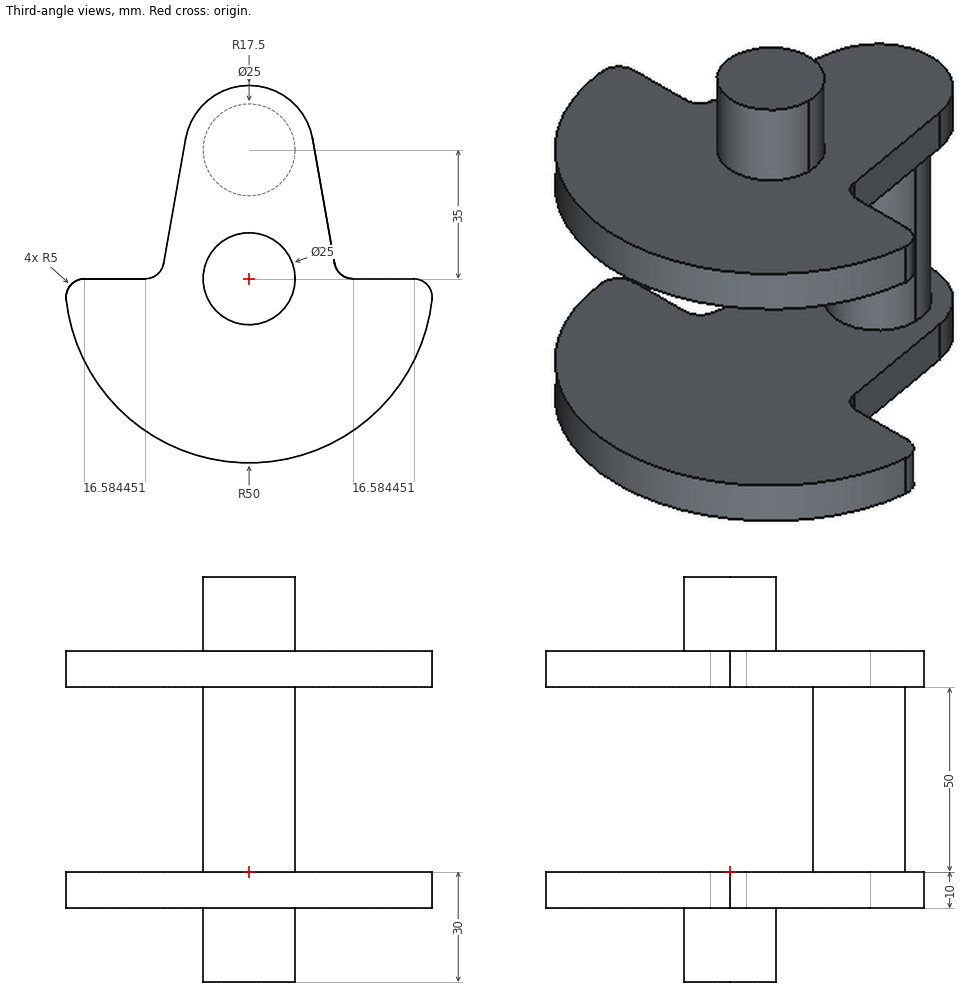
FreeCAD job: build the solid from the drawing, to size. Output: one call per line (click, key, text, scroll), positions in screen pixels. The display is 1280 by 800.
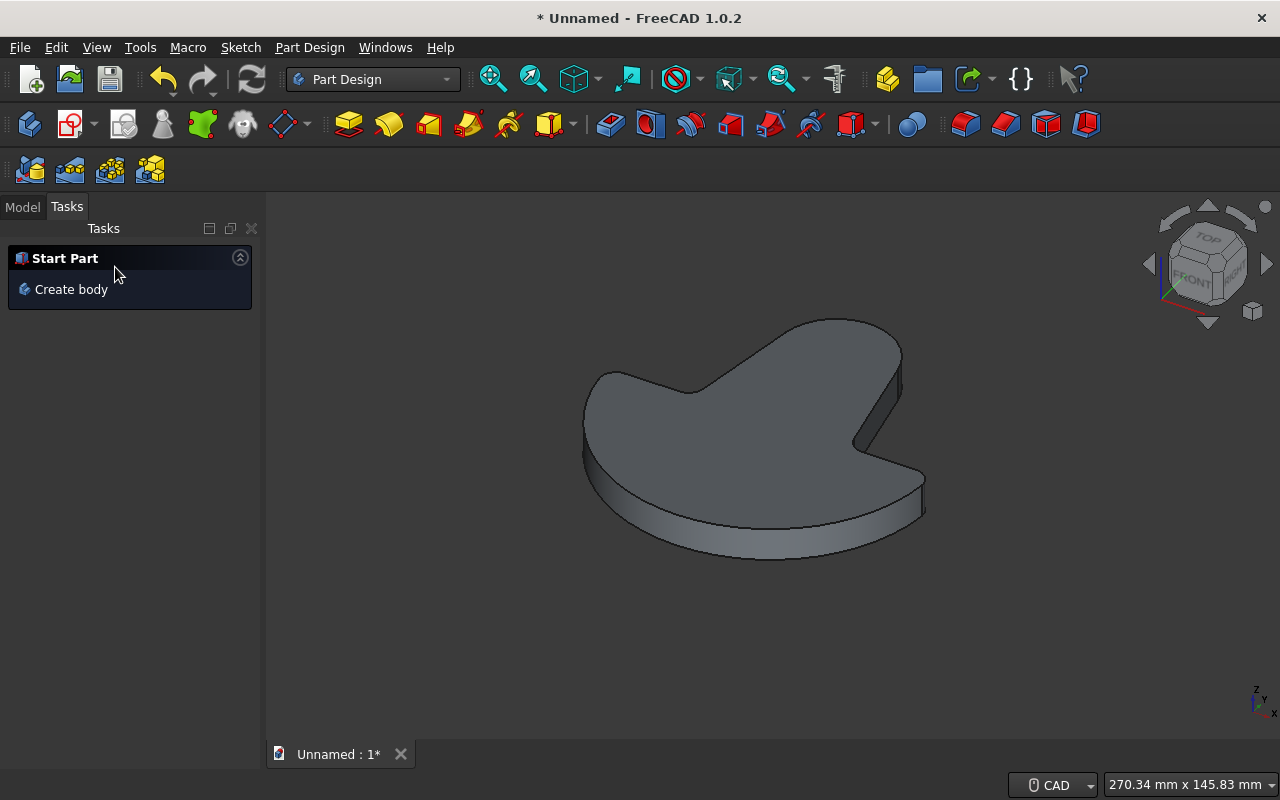
click(70, 124)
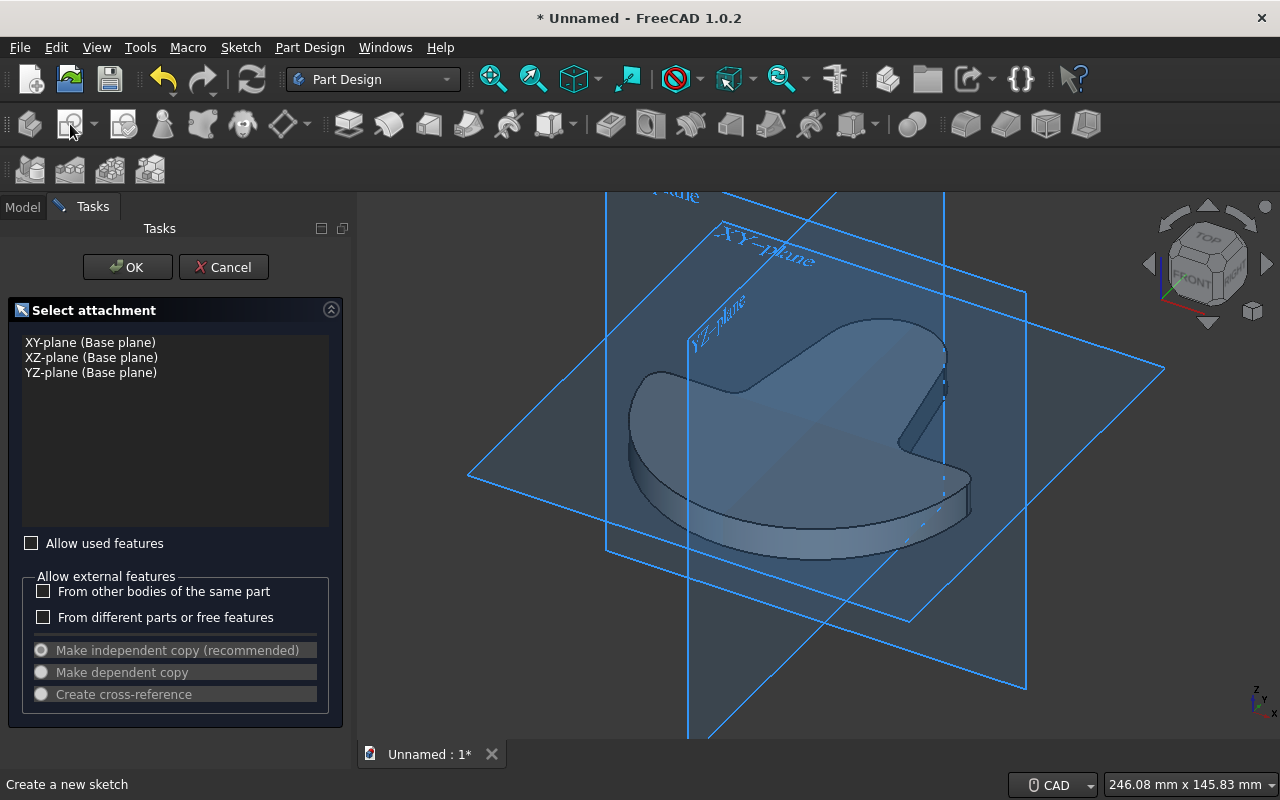
click(82, 342)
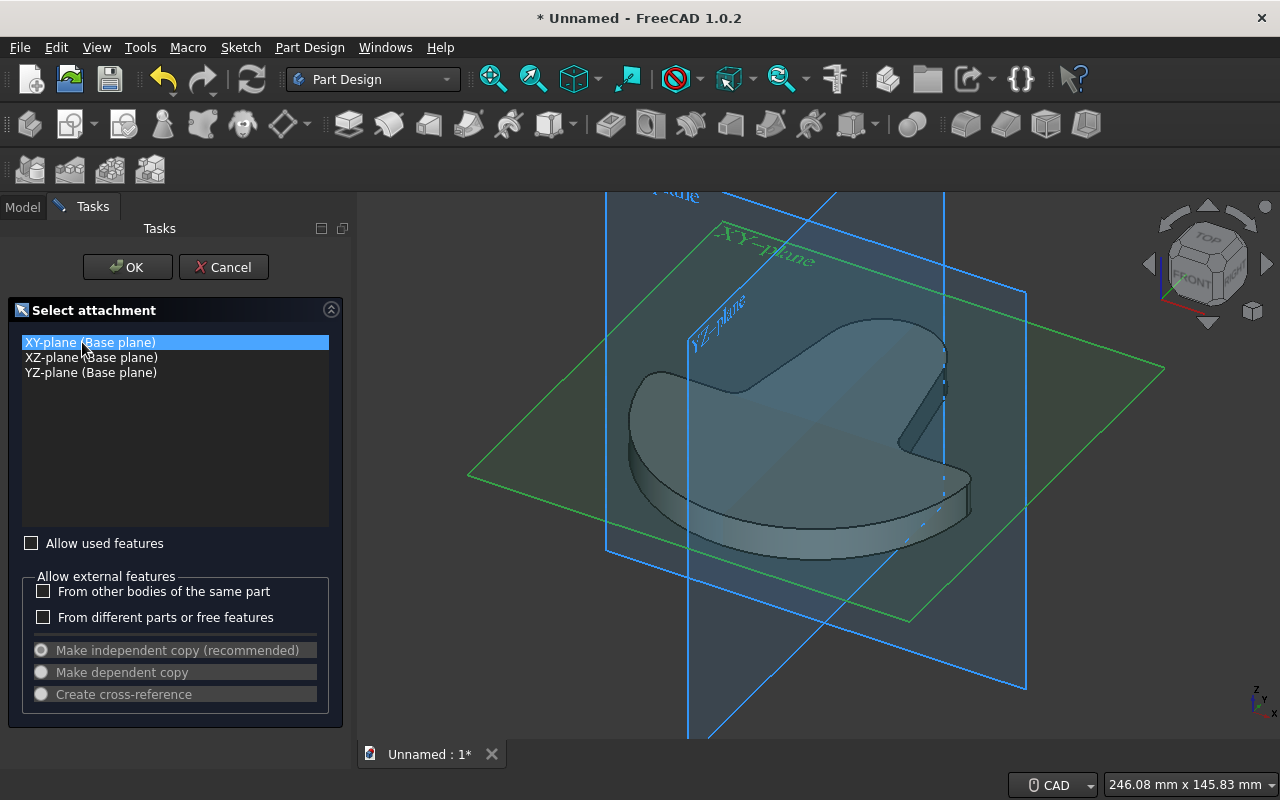
click(128, 267)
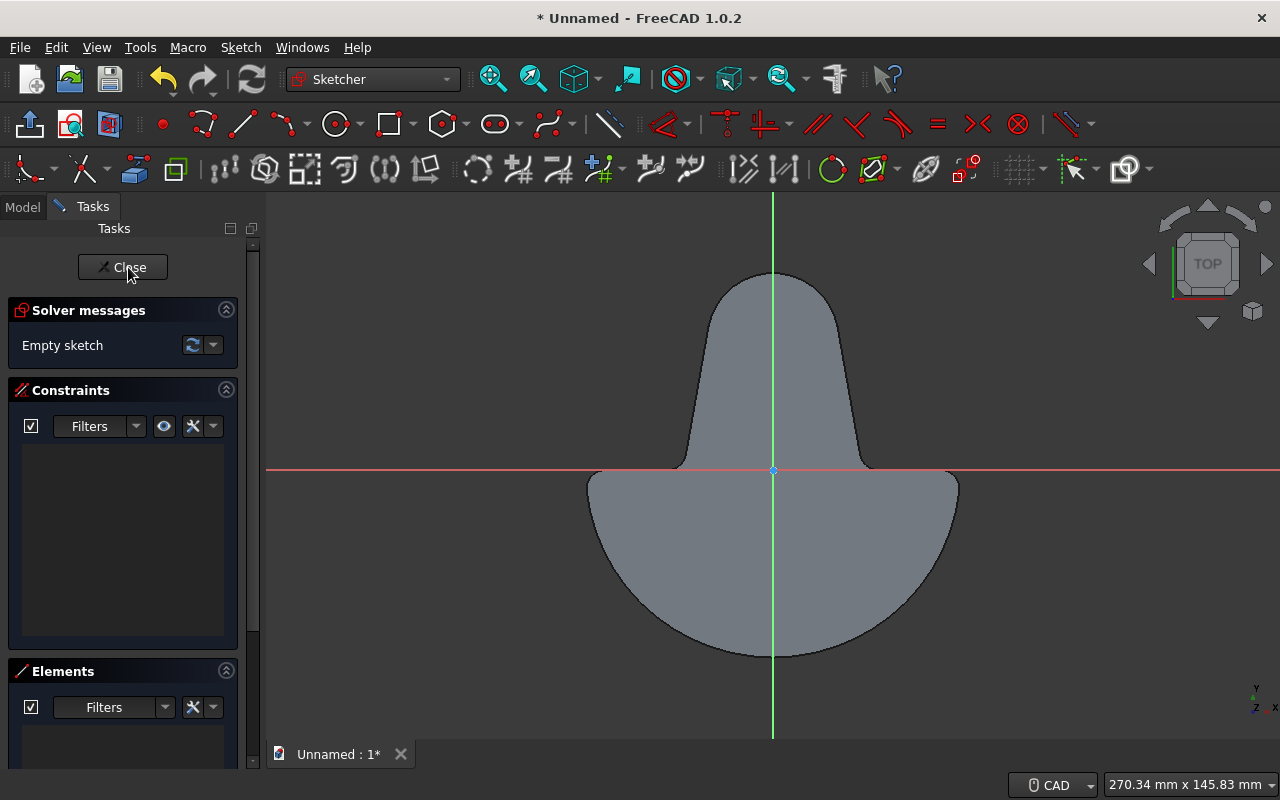
scroll(856, 278, up, 3)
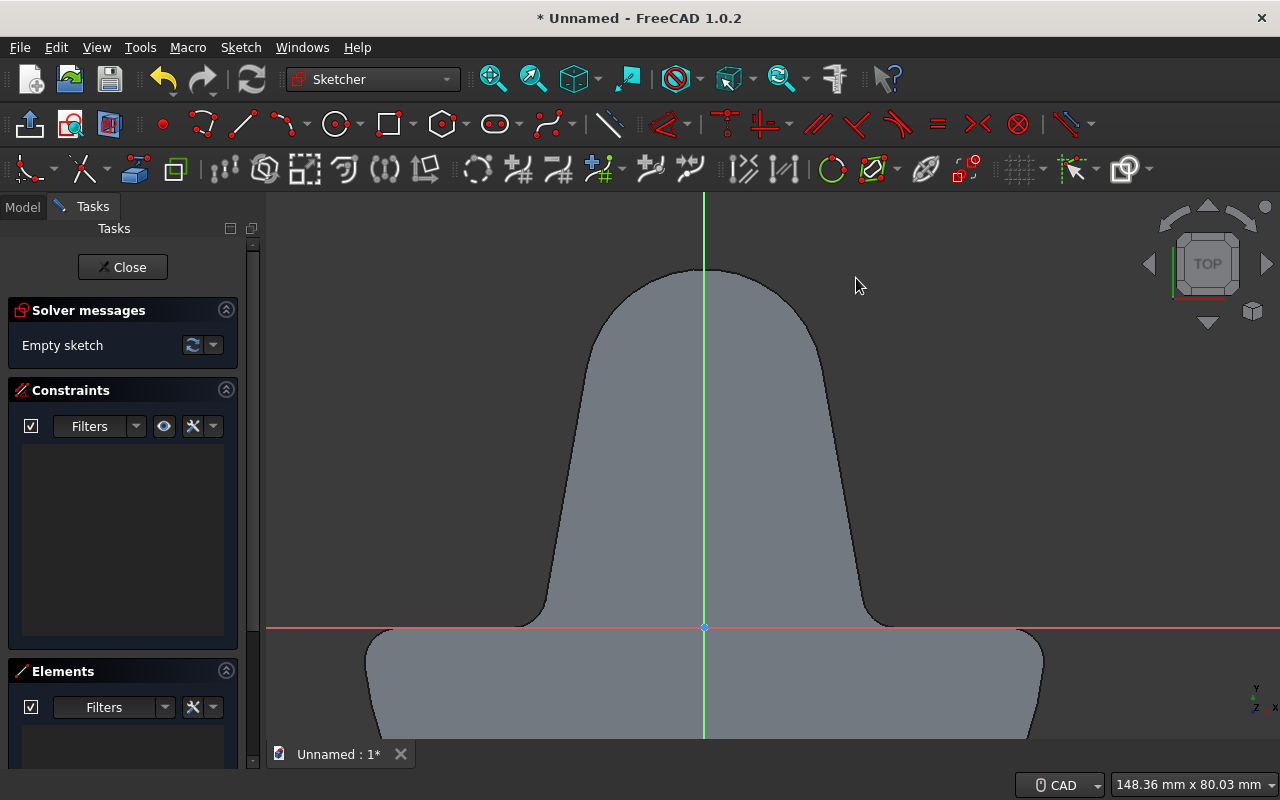
key(g)
key(c)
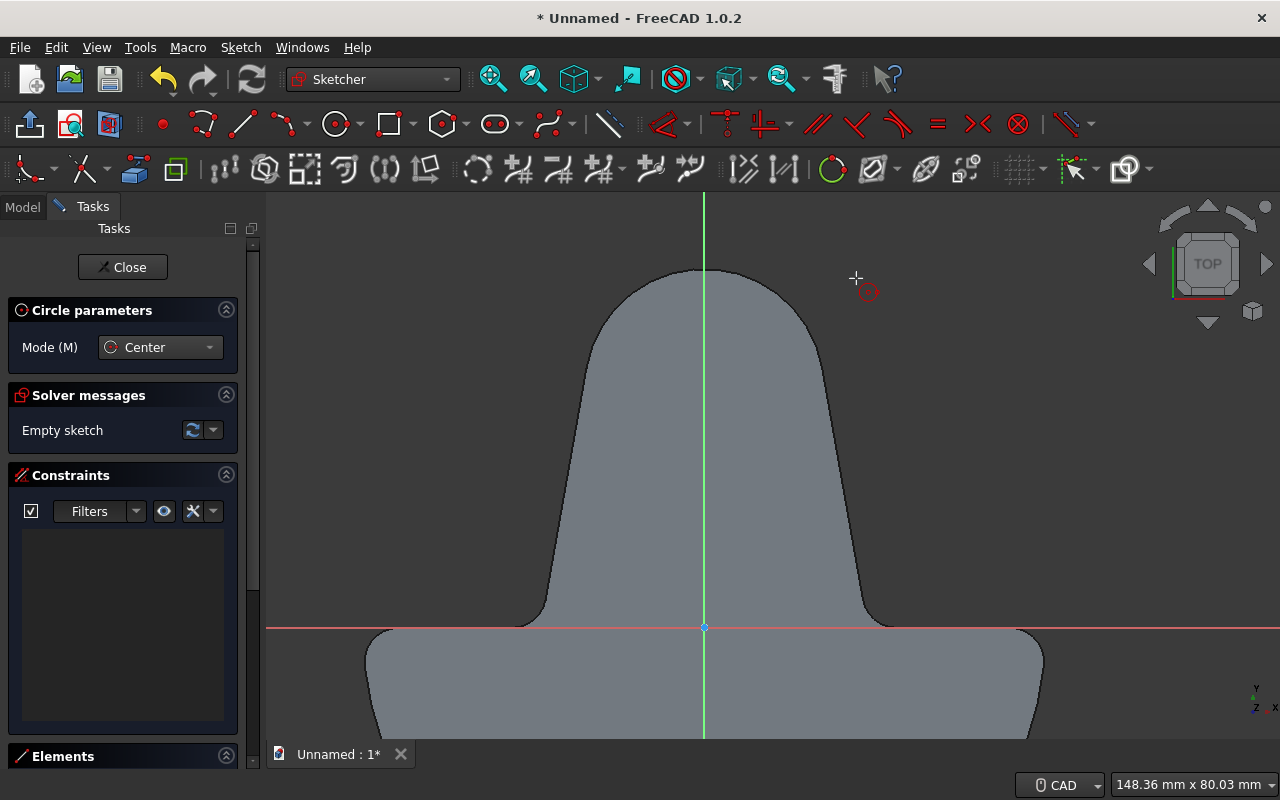
click(704, 389)
click(765, 328)
key(Escape)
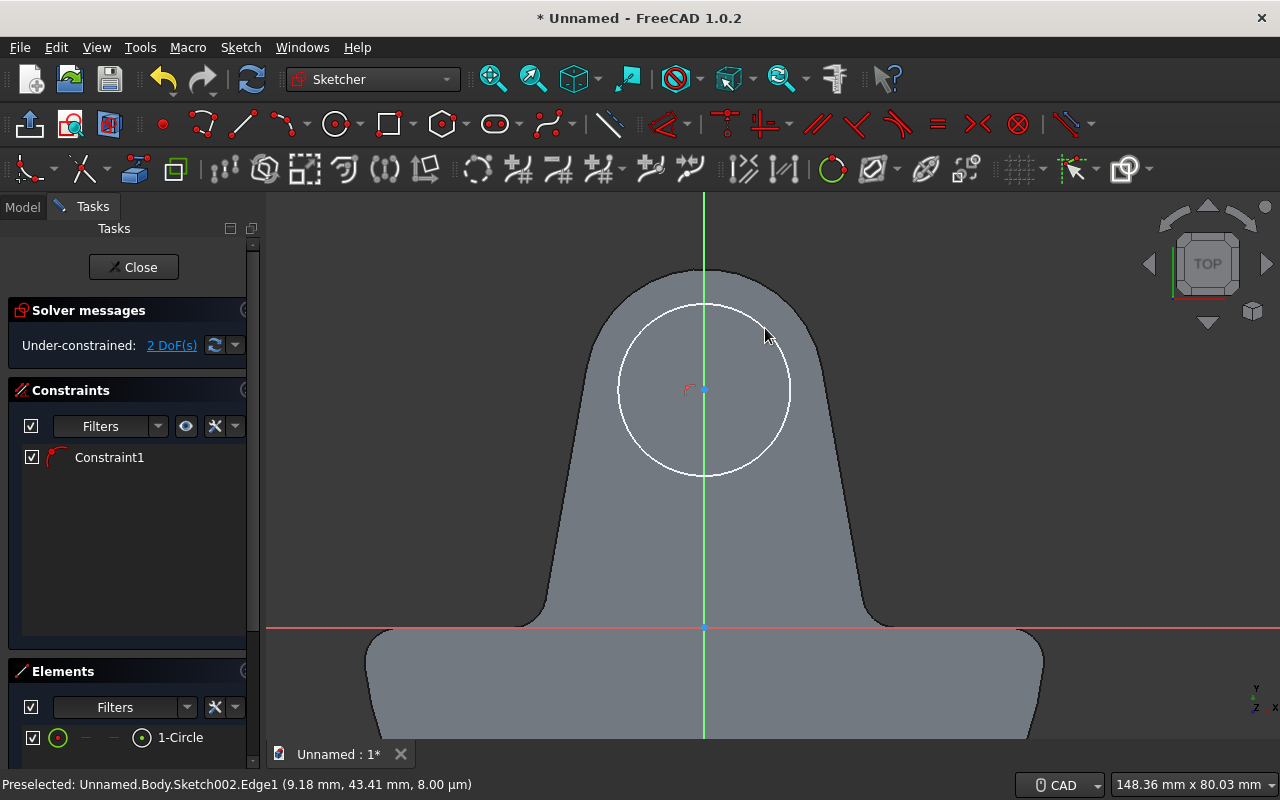
key(d)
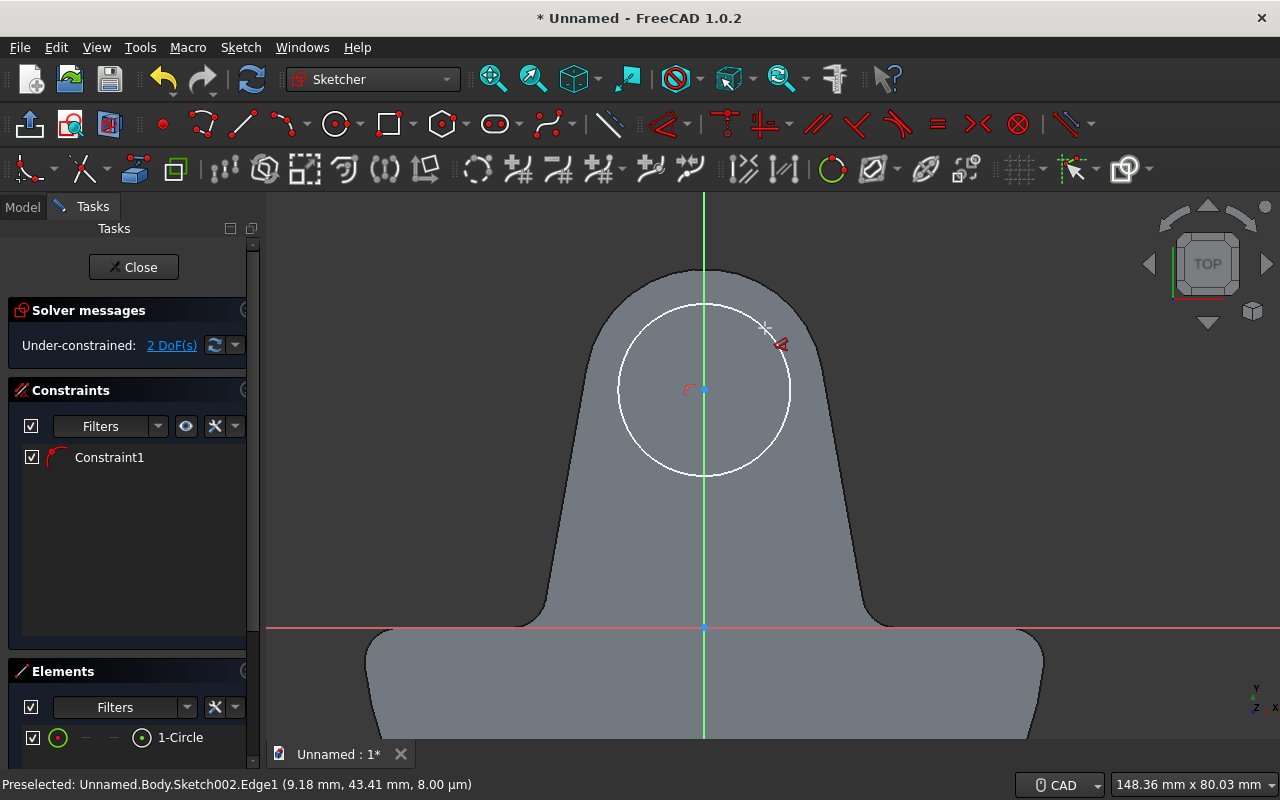
click(765, 329)
click(788, 306)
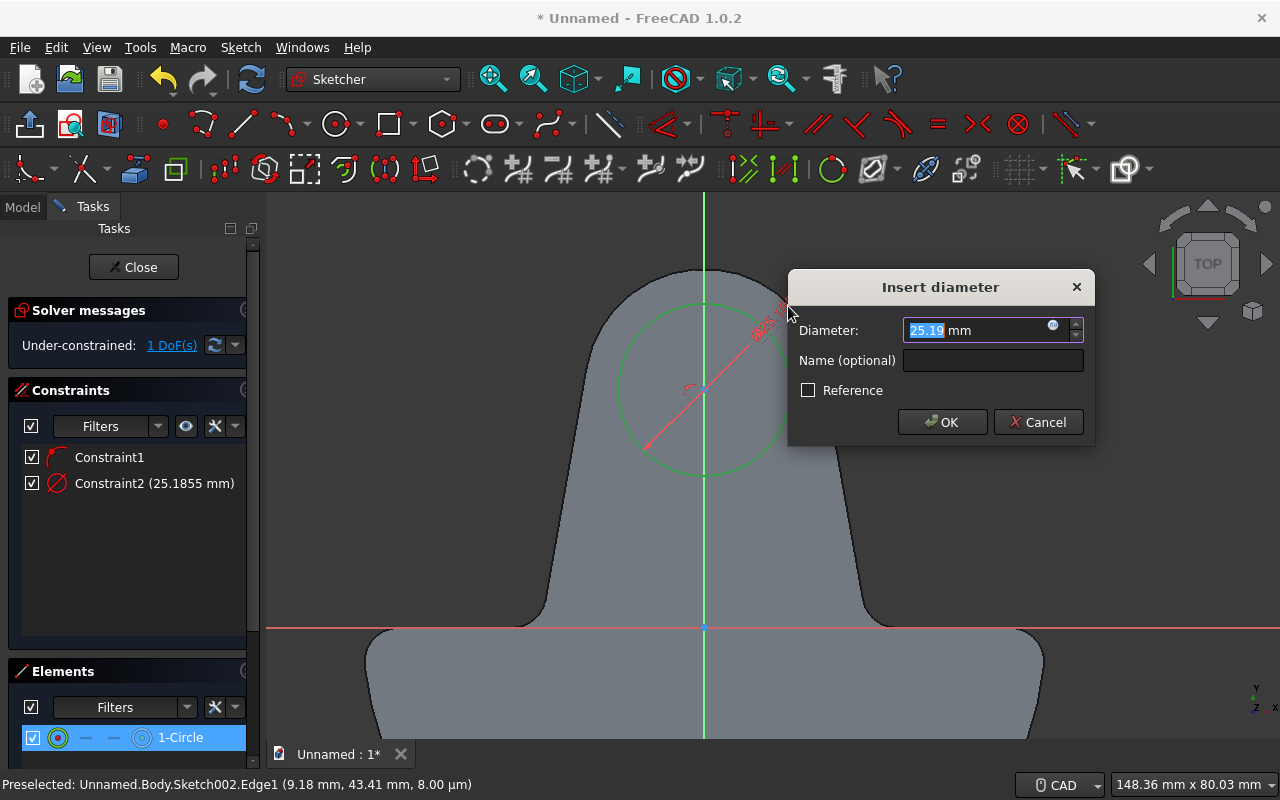
text(25)
key(Return)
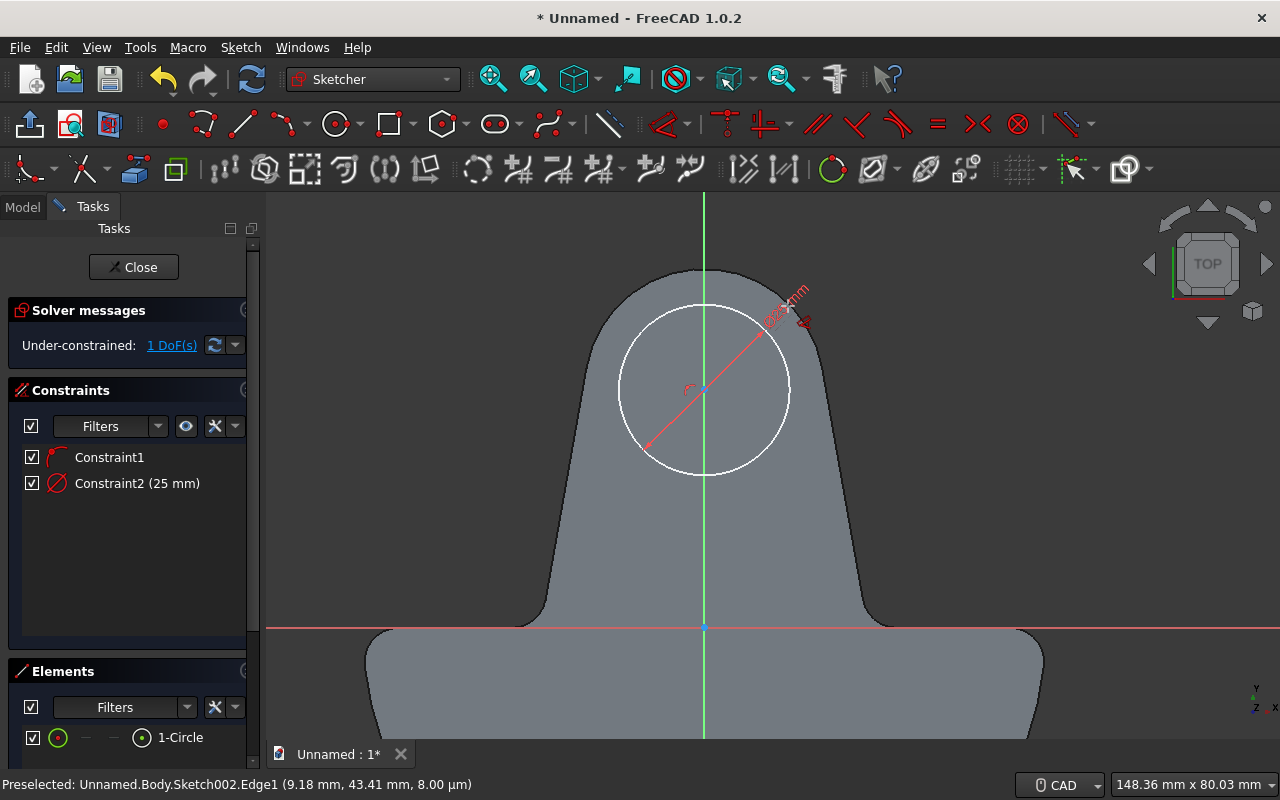
click(704, 390)
click(738, 509)